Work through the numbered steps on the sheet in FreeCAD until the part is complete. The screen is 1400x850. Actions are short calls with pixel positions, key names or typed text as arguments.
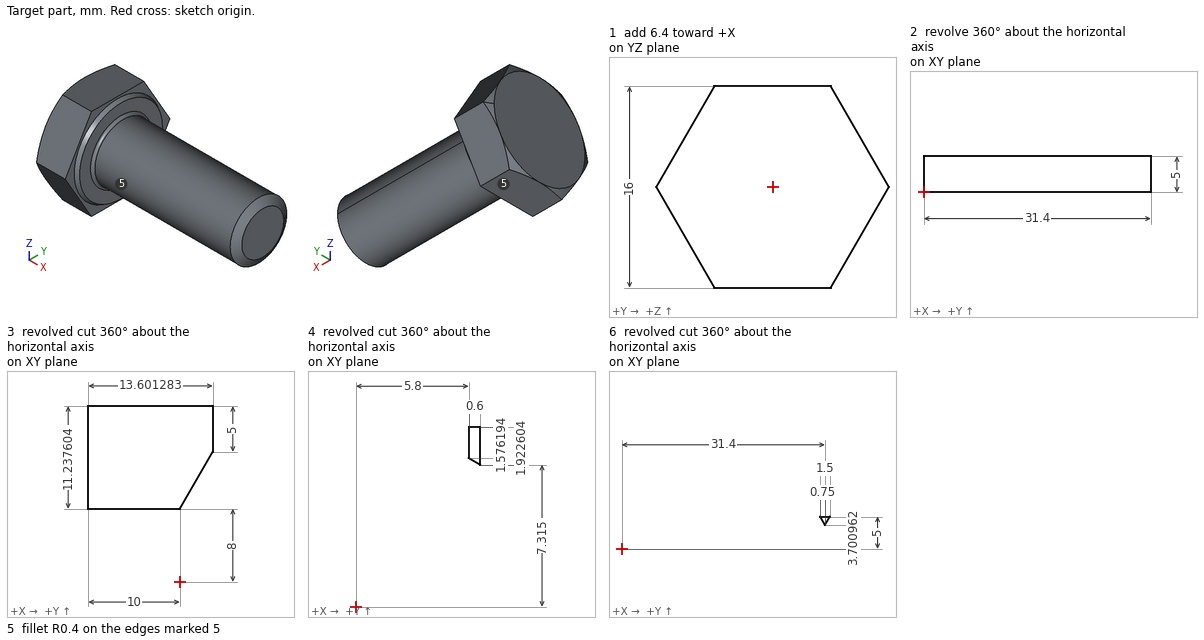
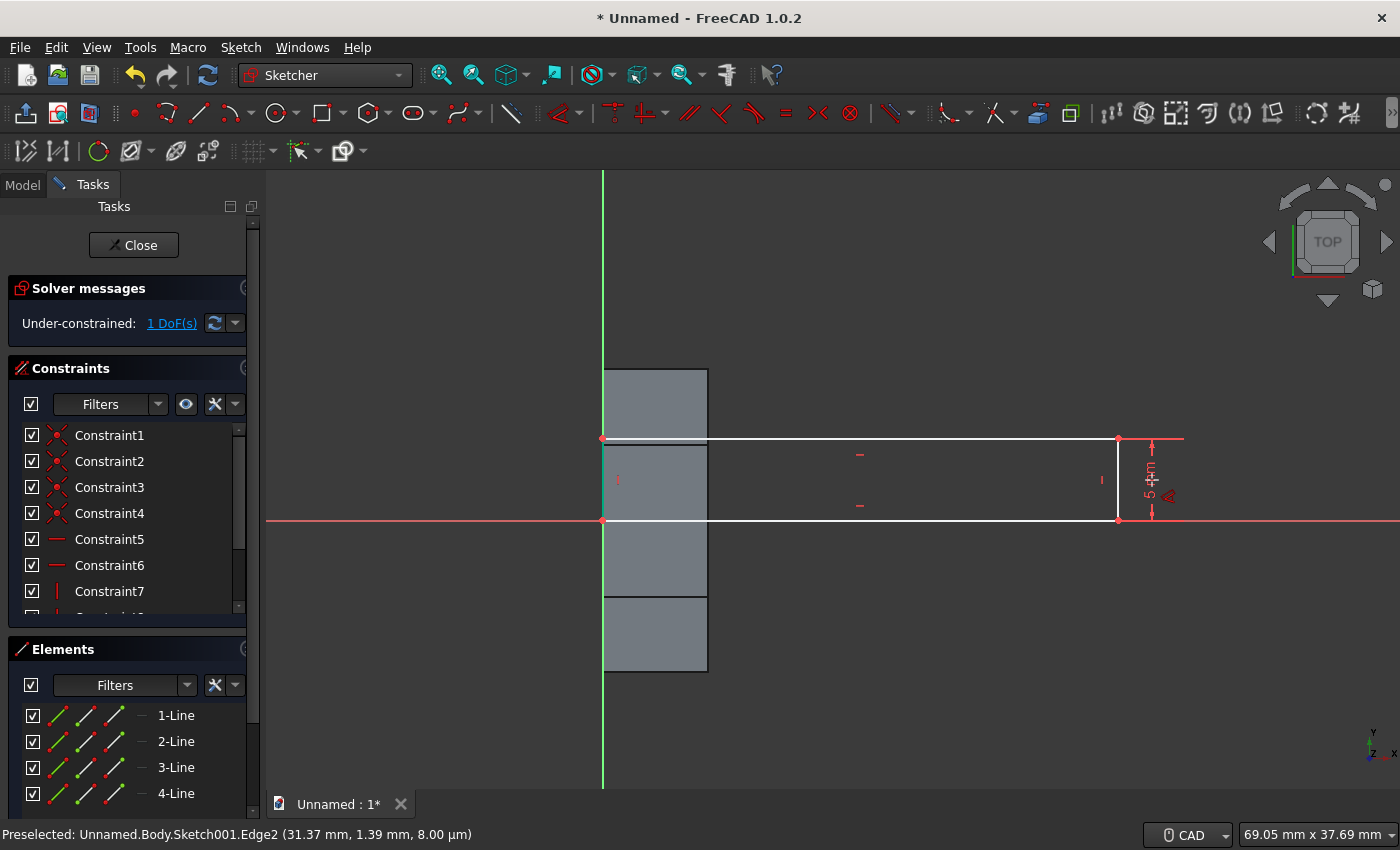
click(757, 521)
click(860, 555)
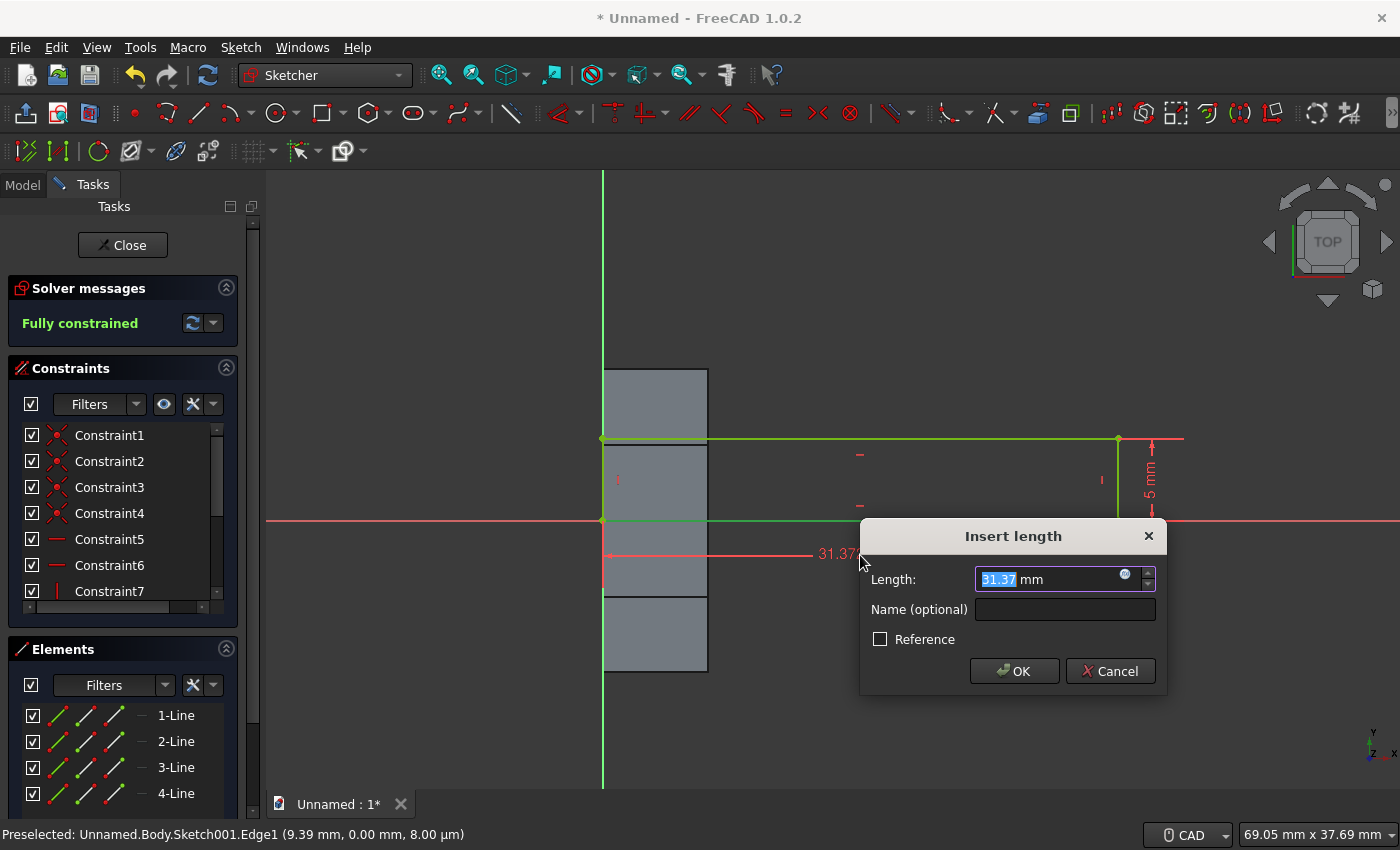
text(31.4)
key(Return)
key(Escape)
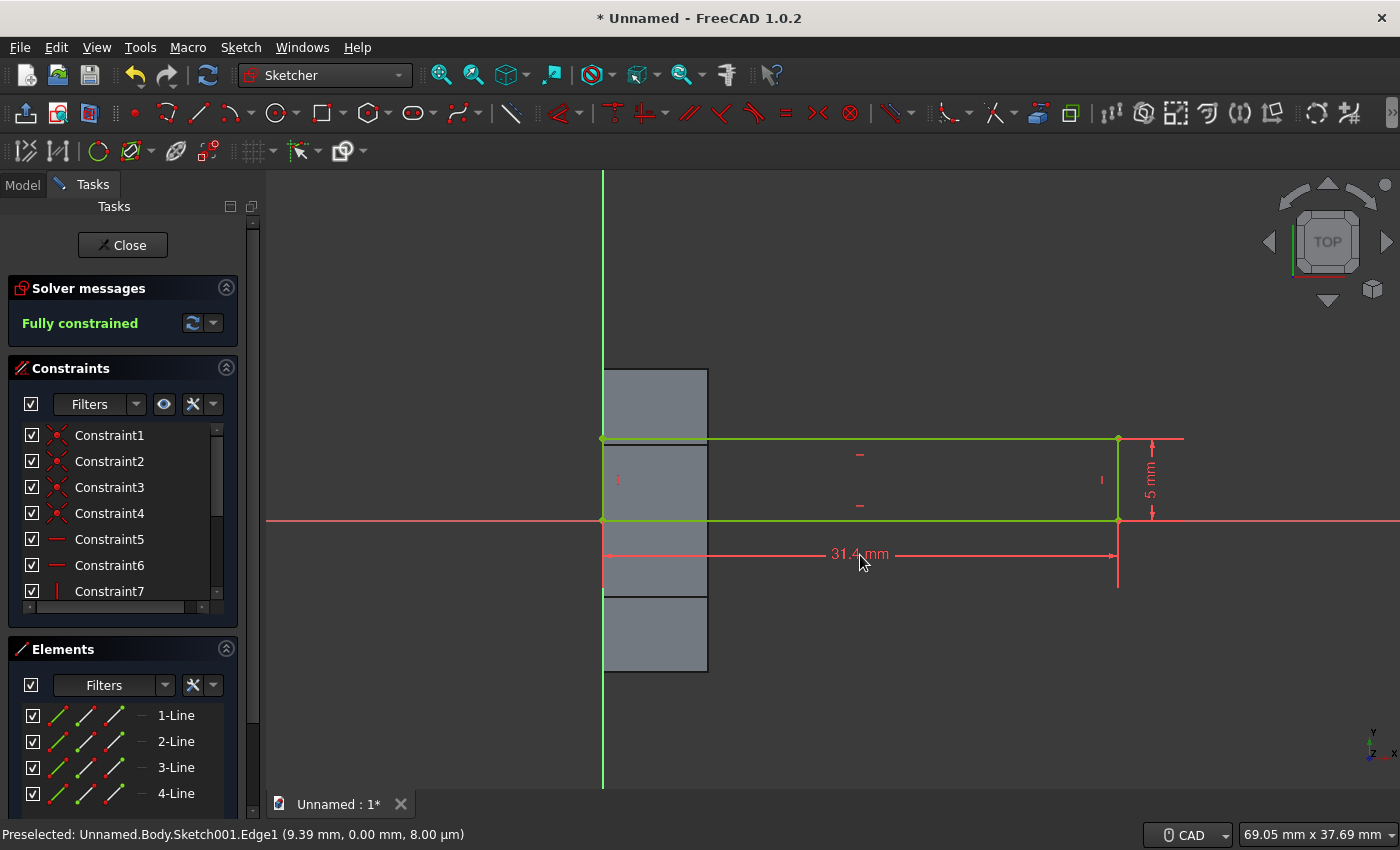
click(123, 245)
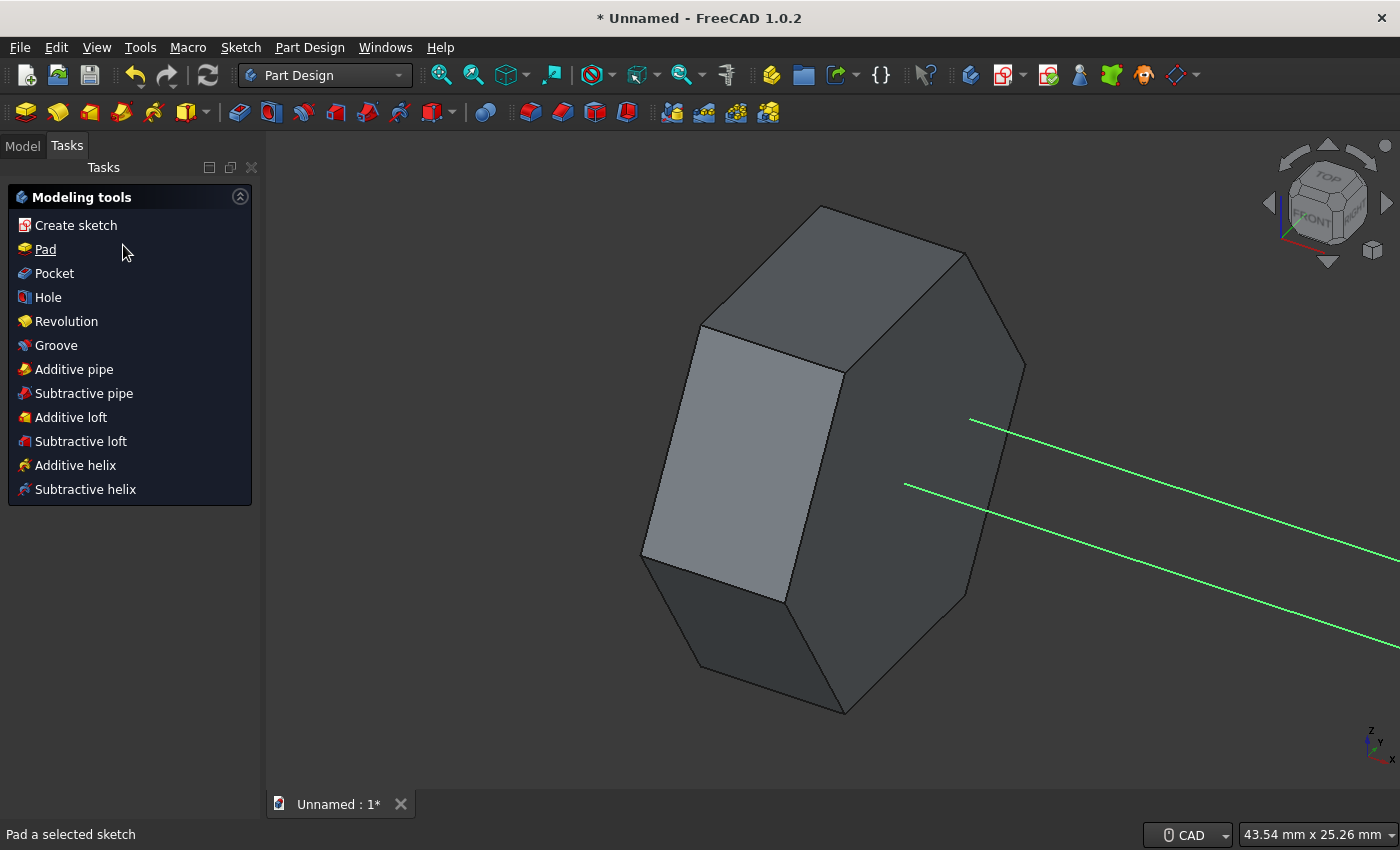
click(58, 112)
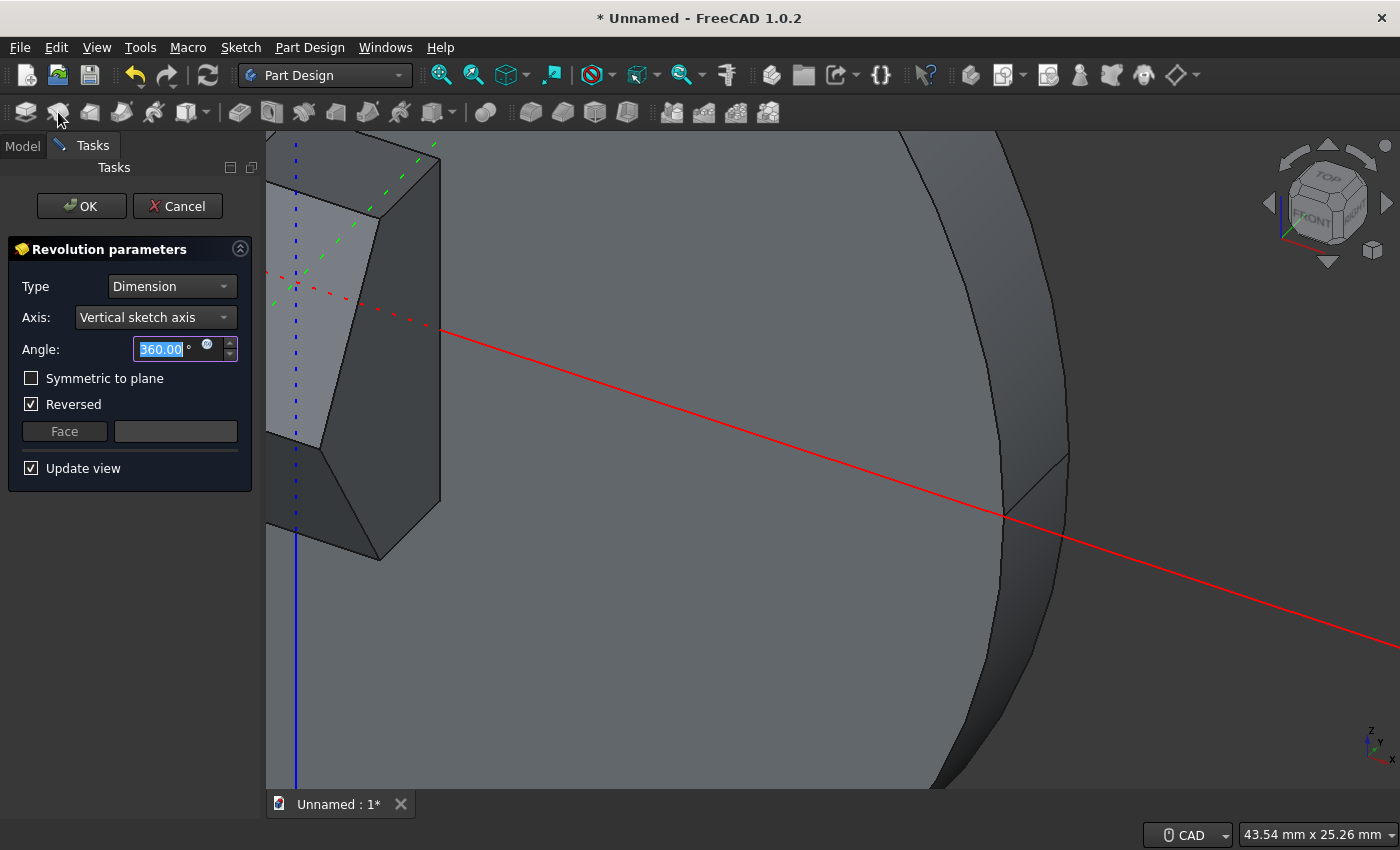
click(156, 318)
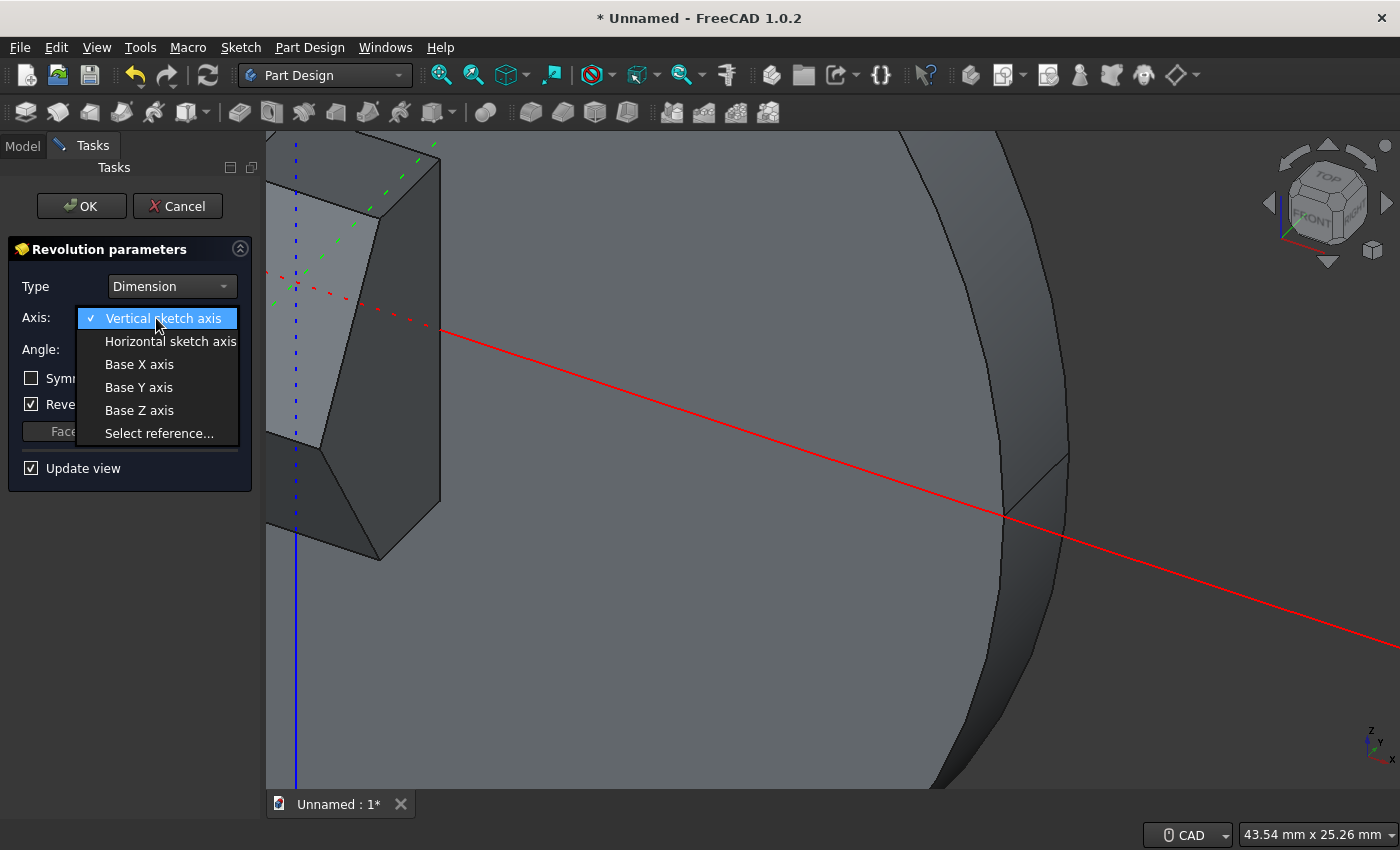
click(156, 342)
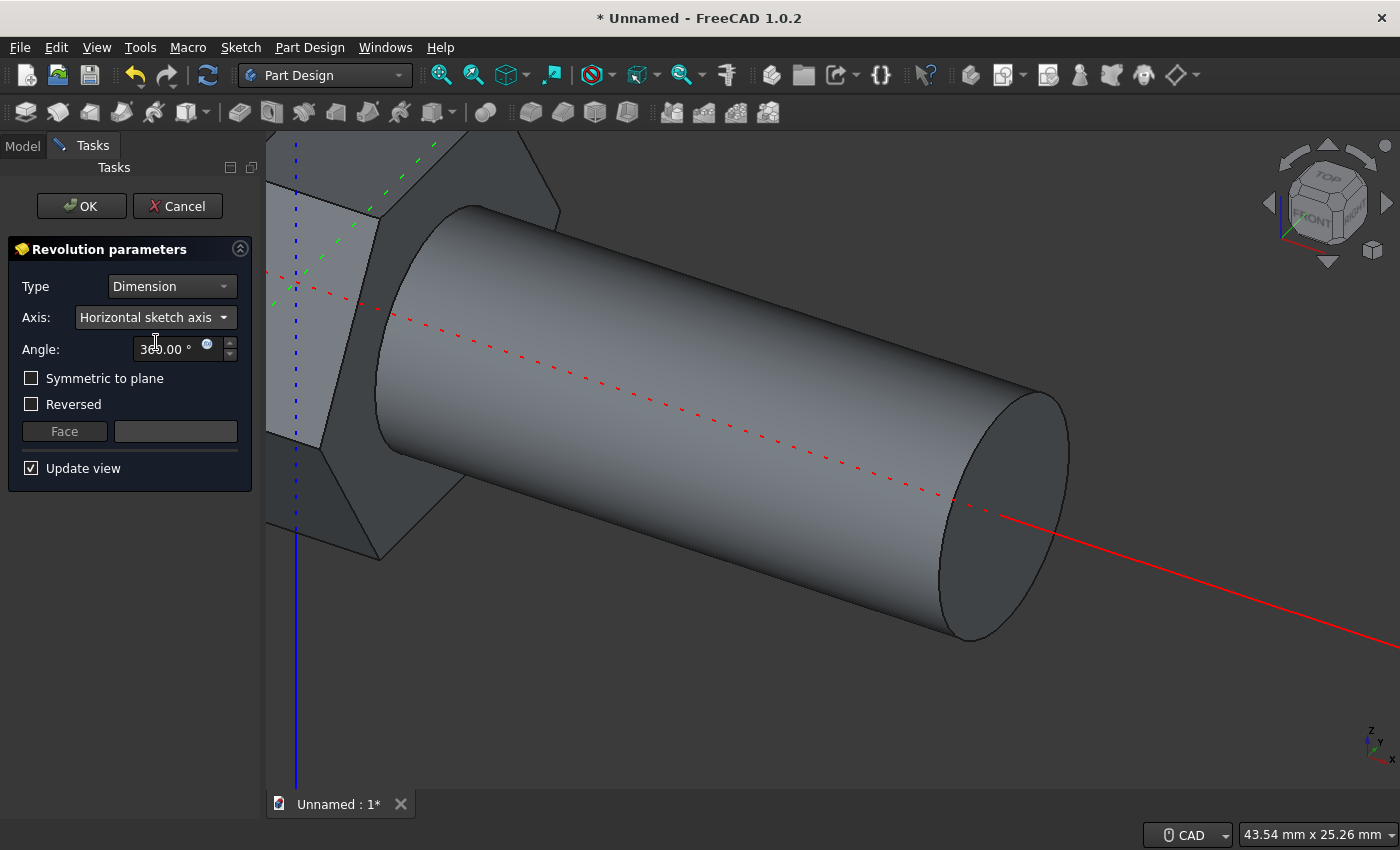
click(82, 206)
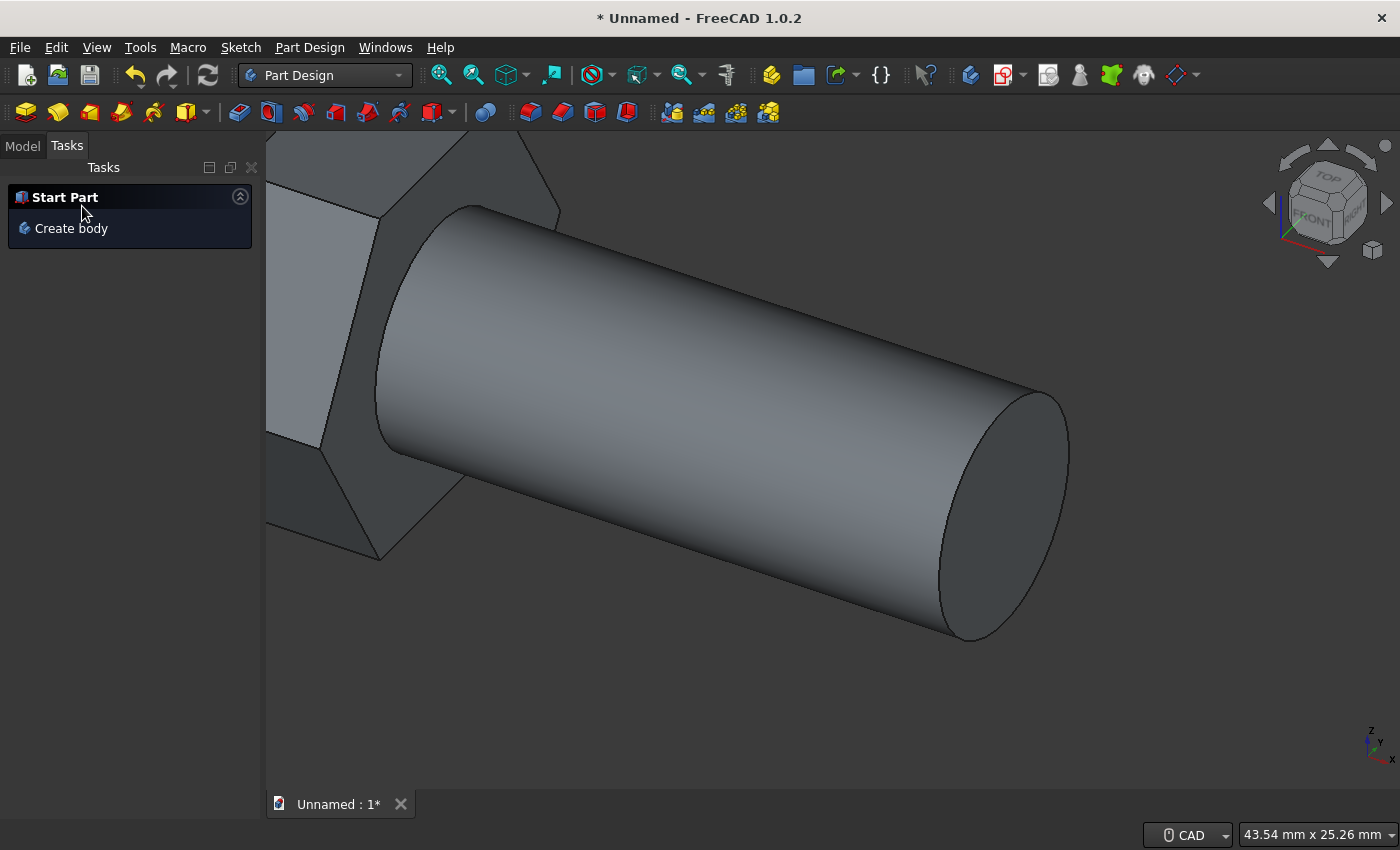
key(v)
key(f)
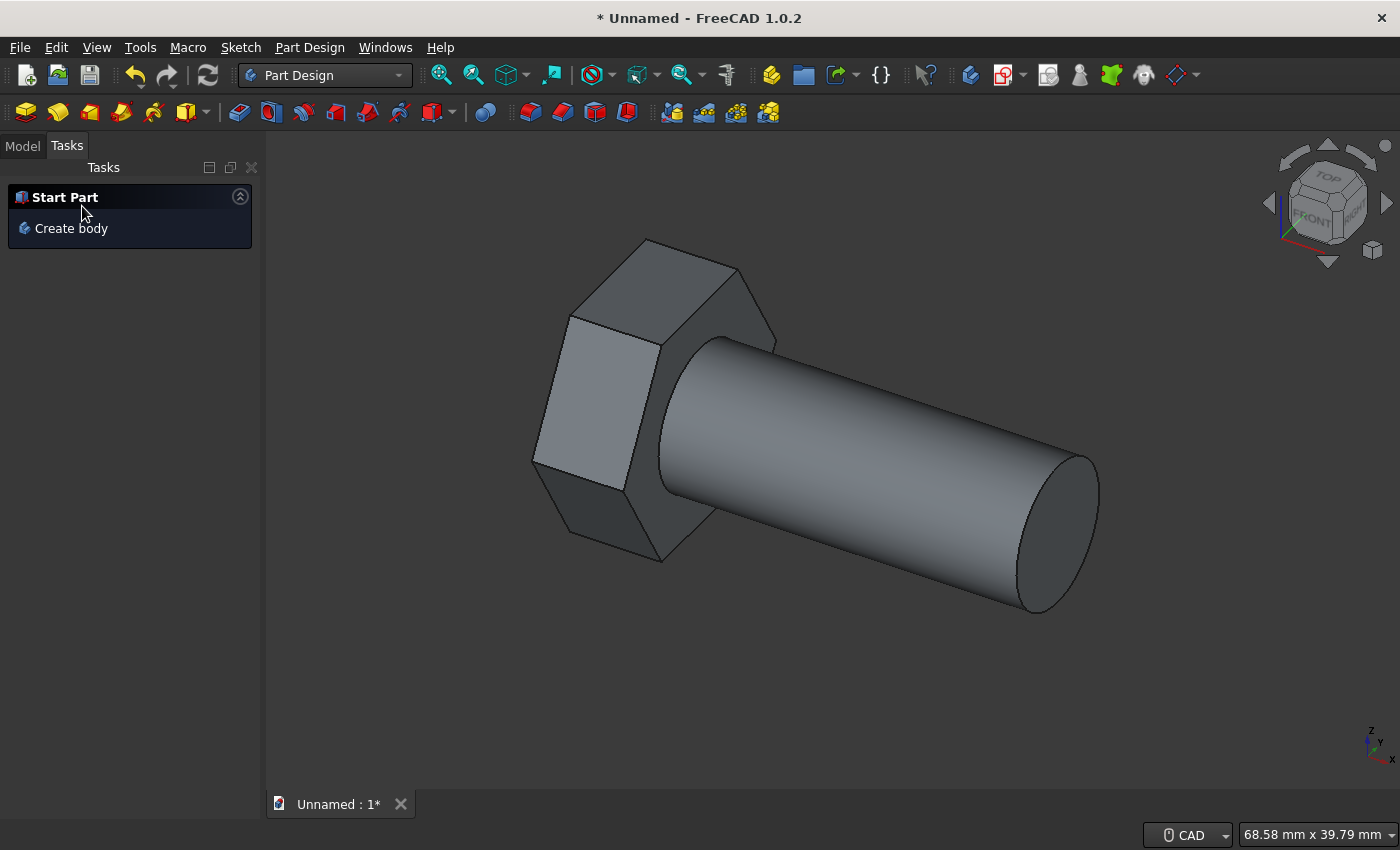
click(1004, 76)